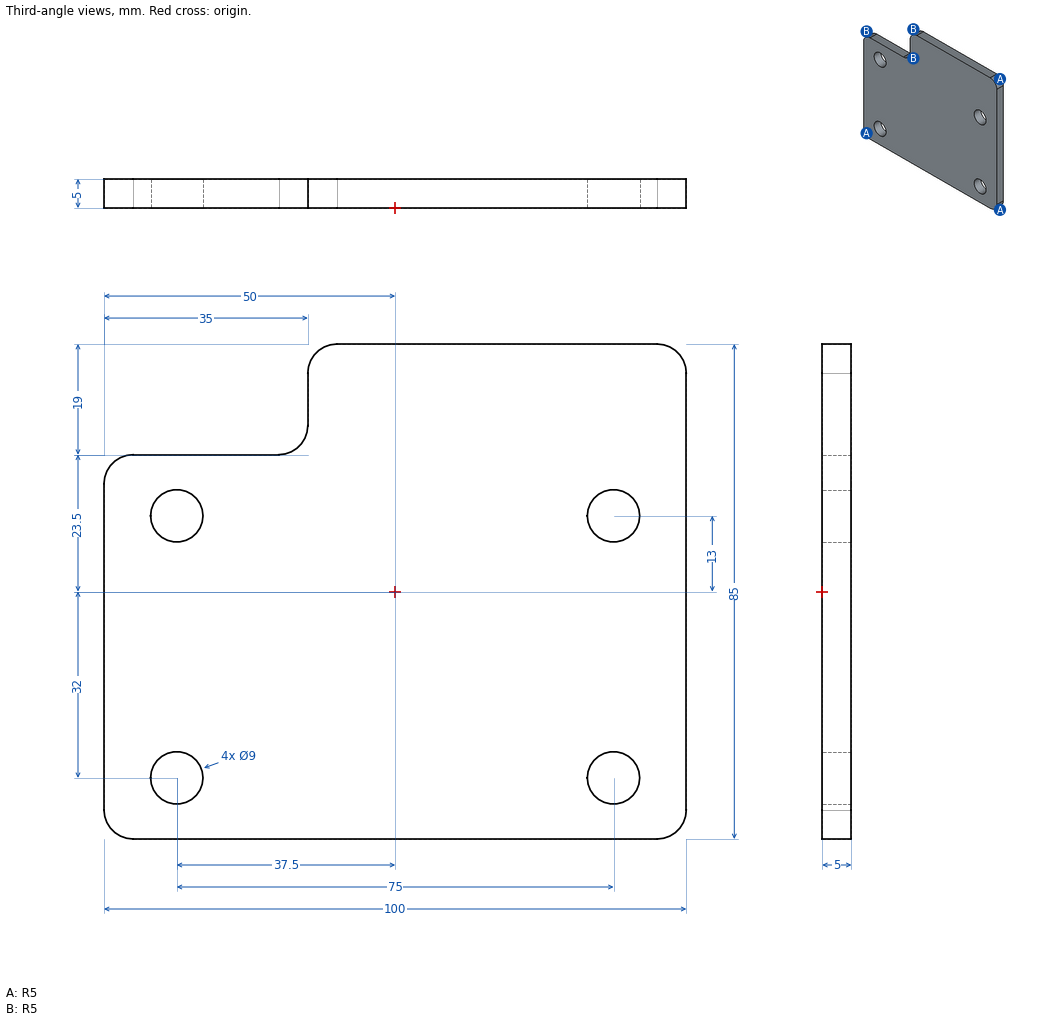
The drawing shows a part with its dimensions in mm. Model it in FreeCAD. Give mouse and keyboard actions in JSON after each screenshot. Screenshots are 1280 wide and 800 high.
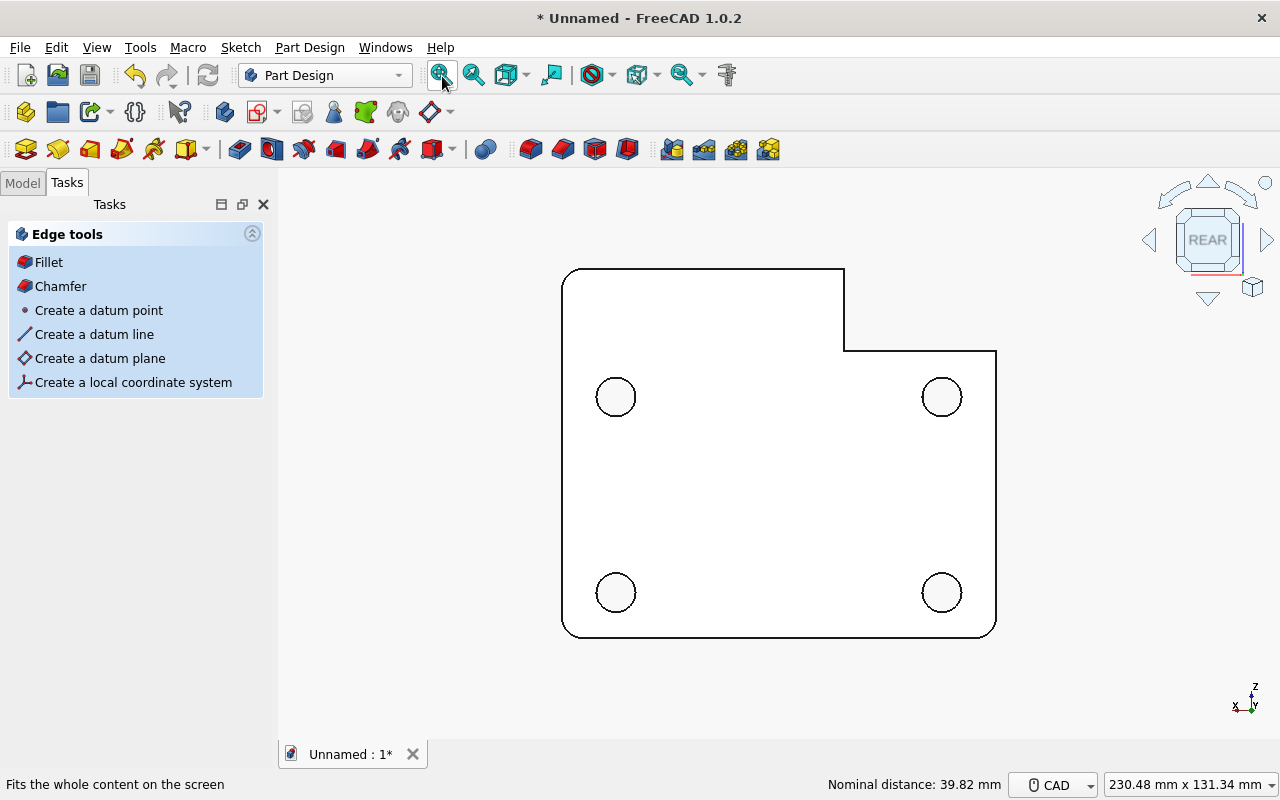
{"action": "scroll", "coordinate": [844, 350], "scroll_direction": "up", "scroll_amount": 4}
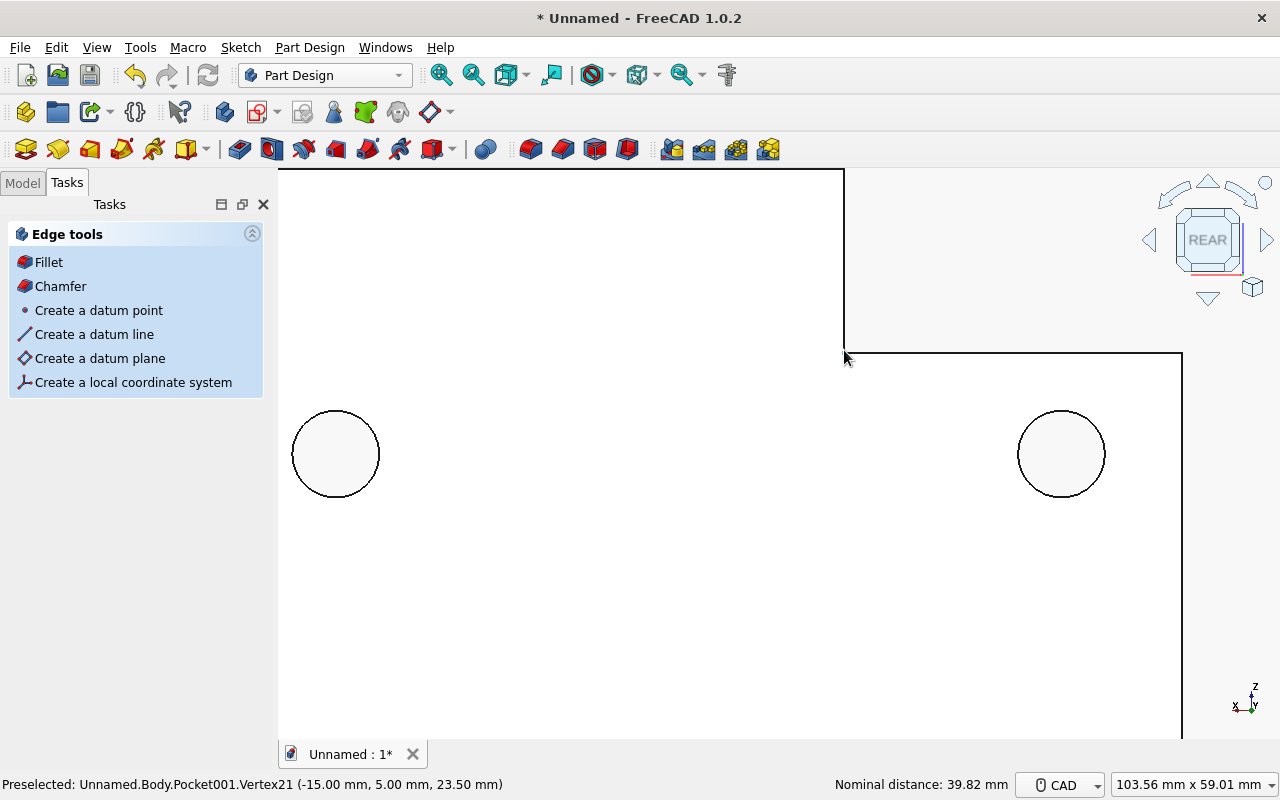
{"action": "key", "text": "v f"}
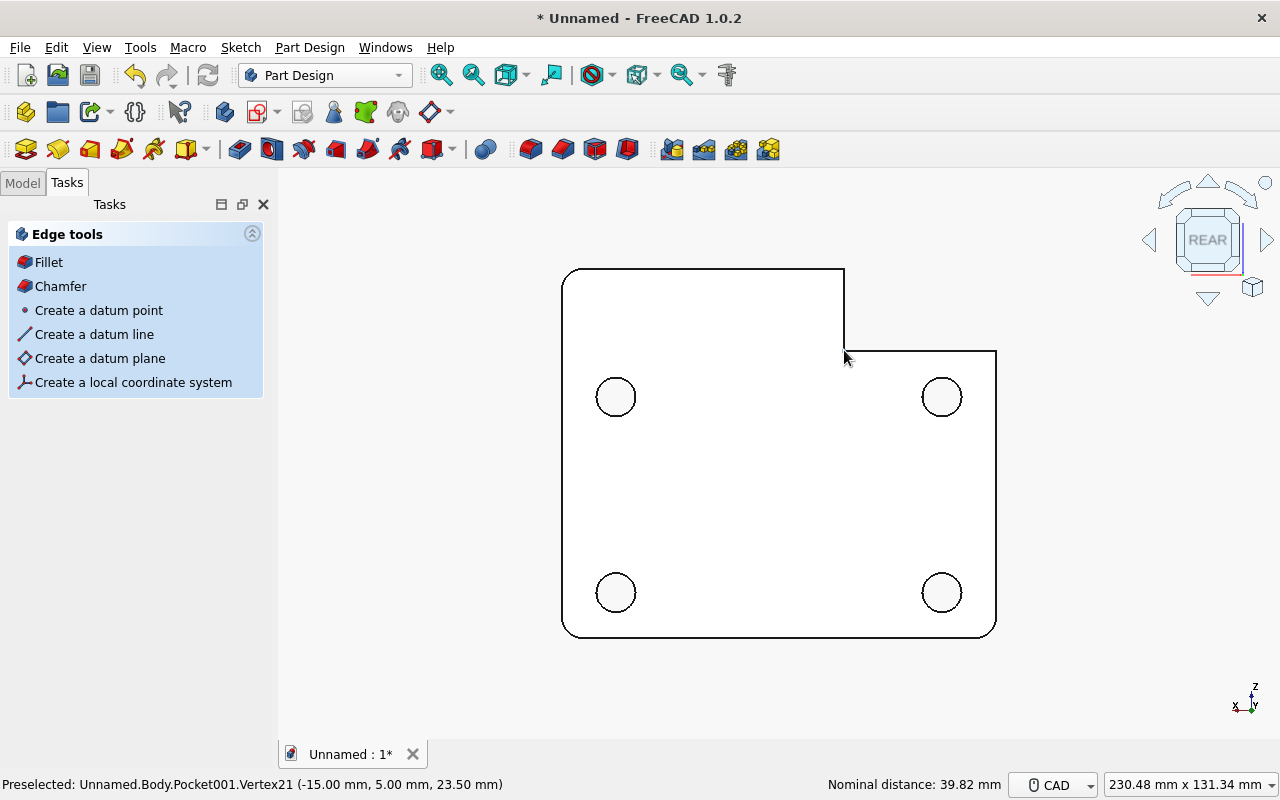
{"action": "key", "text": "6"}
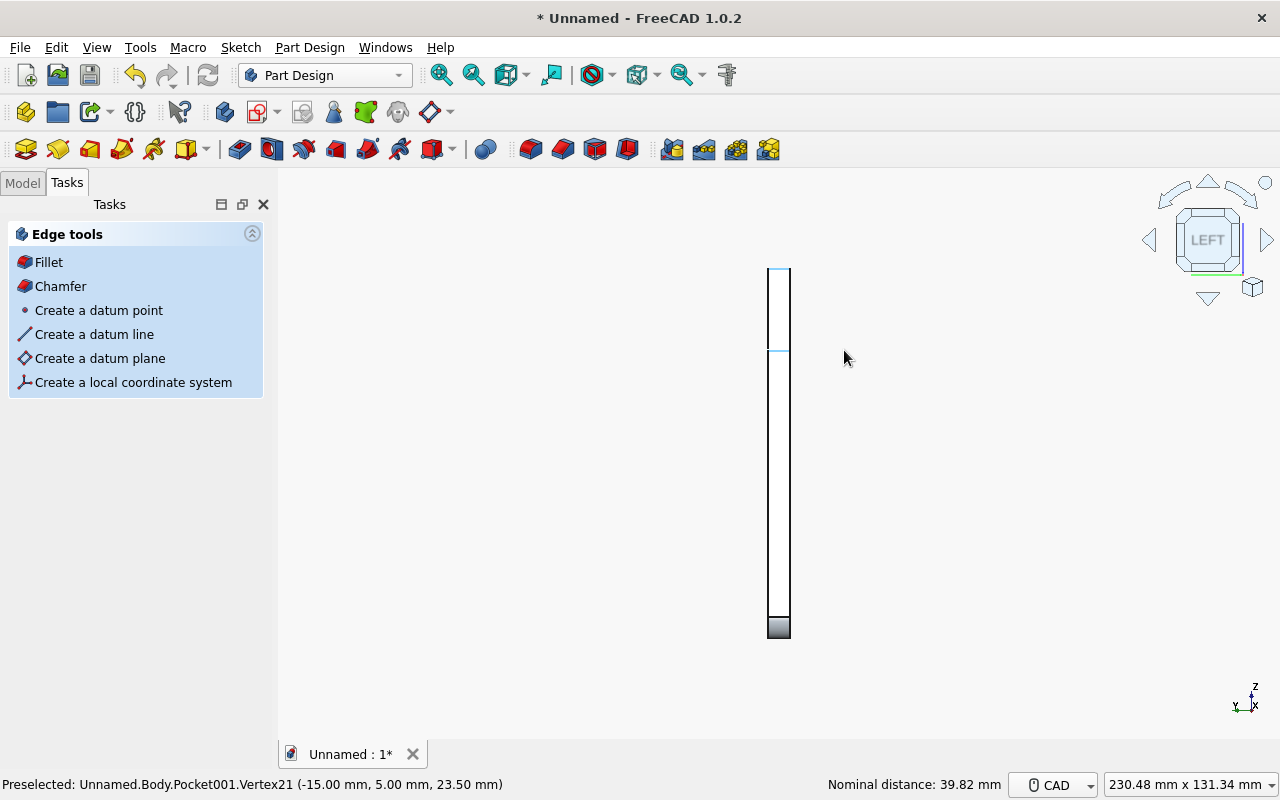
{"action": "scroll", "coordinate": [779, 350], "scroll_direction": "up", "scroll_amount": 4}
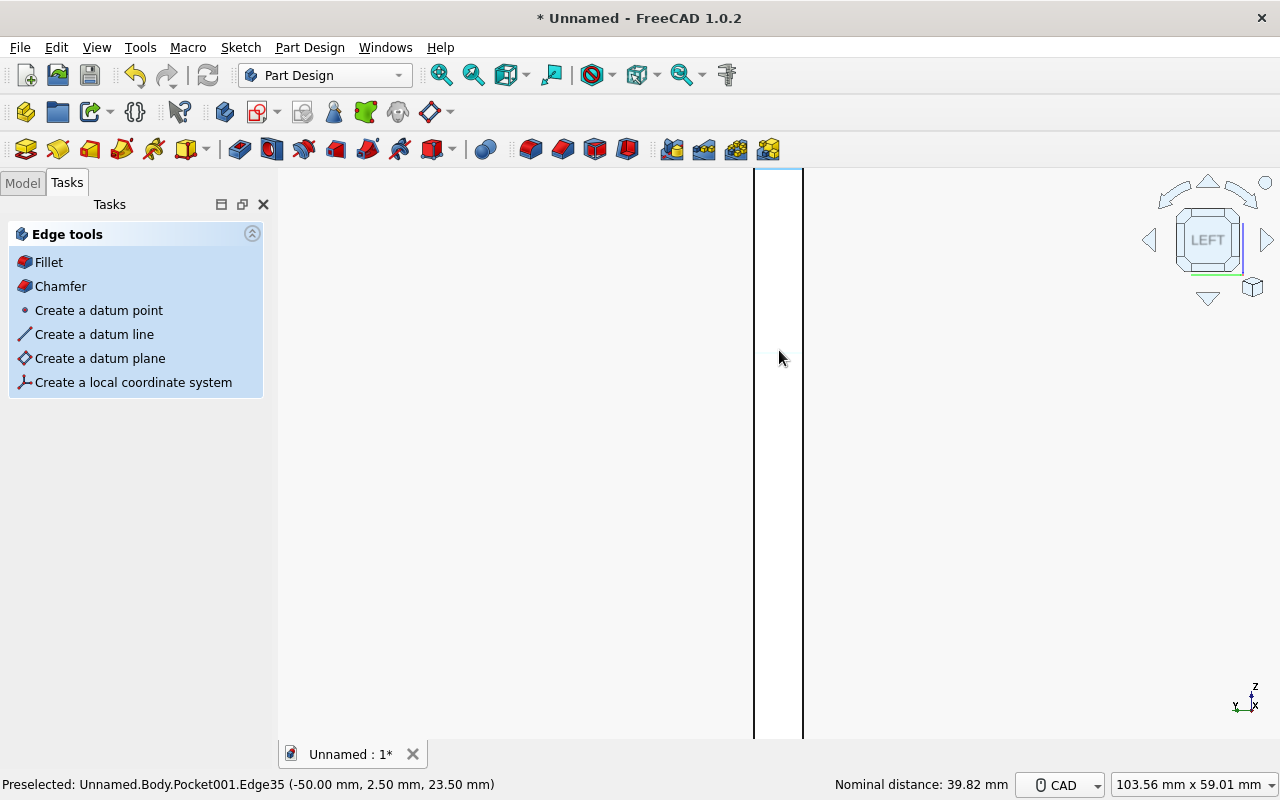
{"action": "key", "text": "v f"}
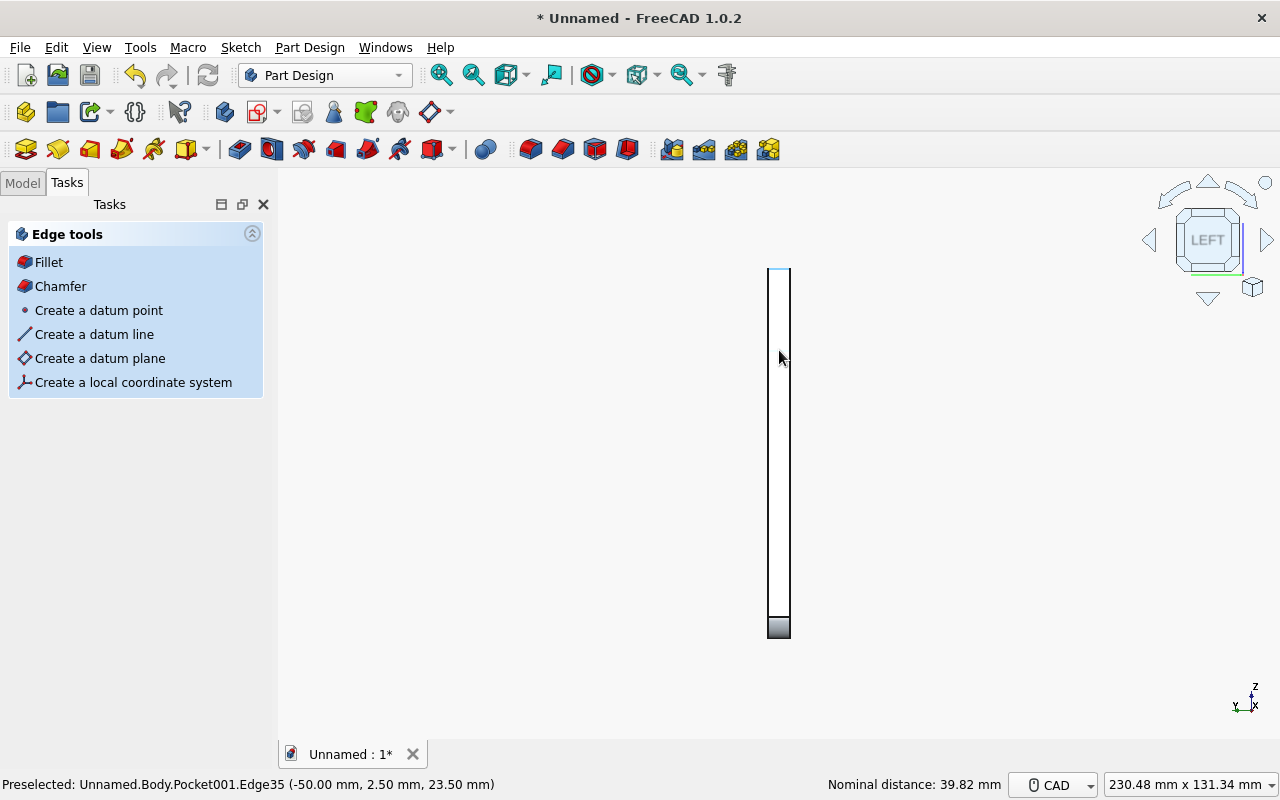
{"action": "key", "text": "v 3"}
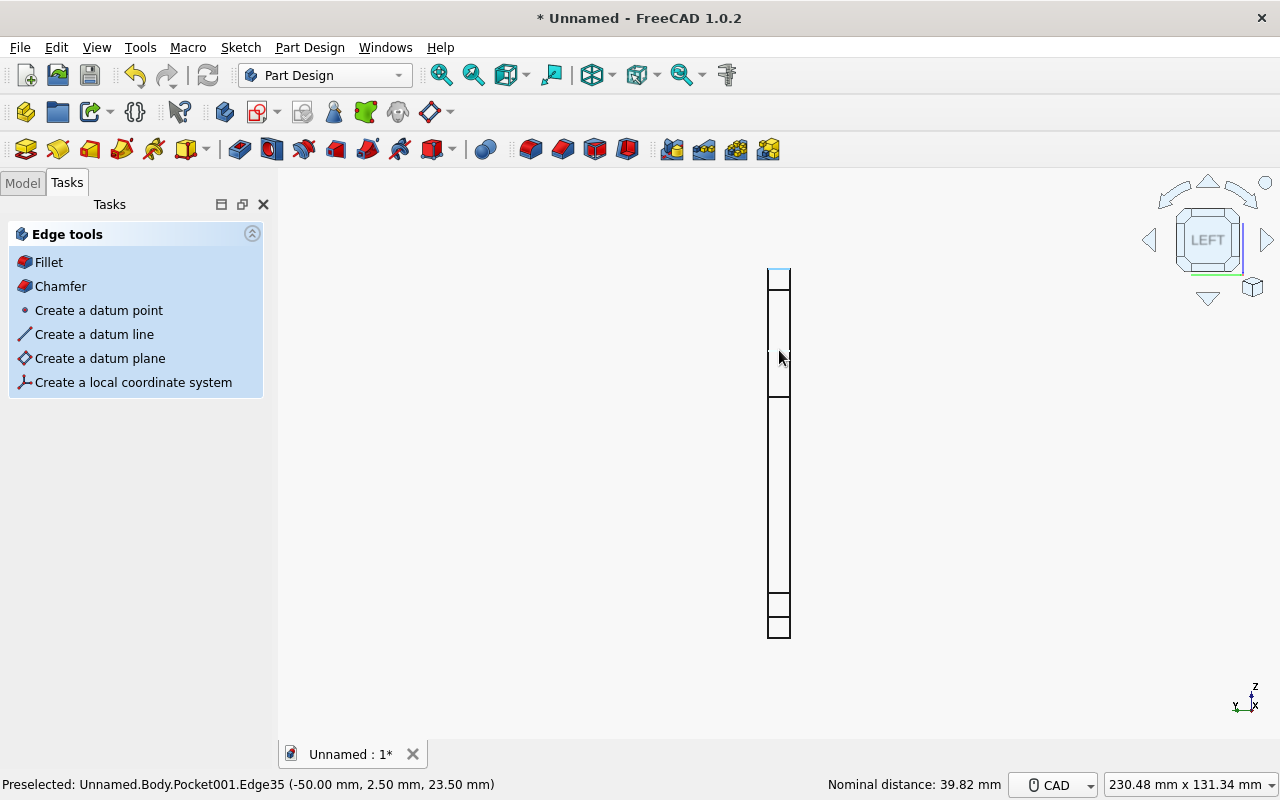
{"action": "key", "text": "0"}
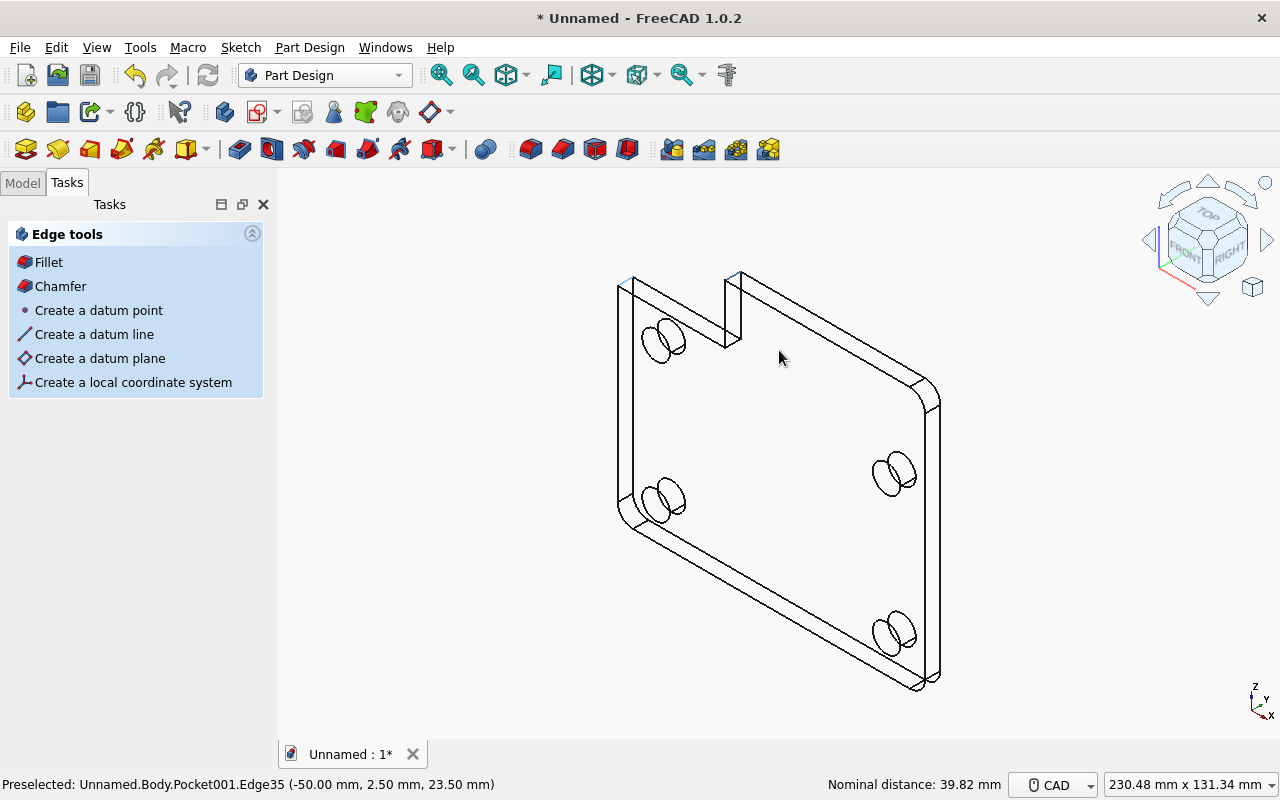
{"action": "left_click", "coordinate": [733, 342], "text": "ctrl"}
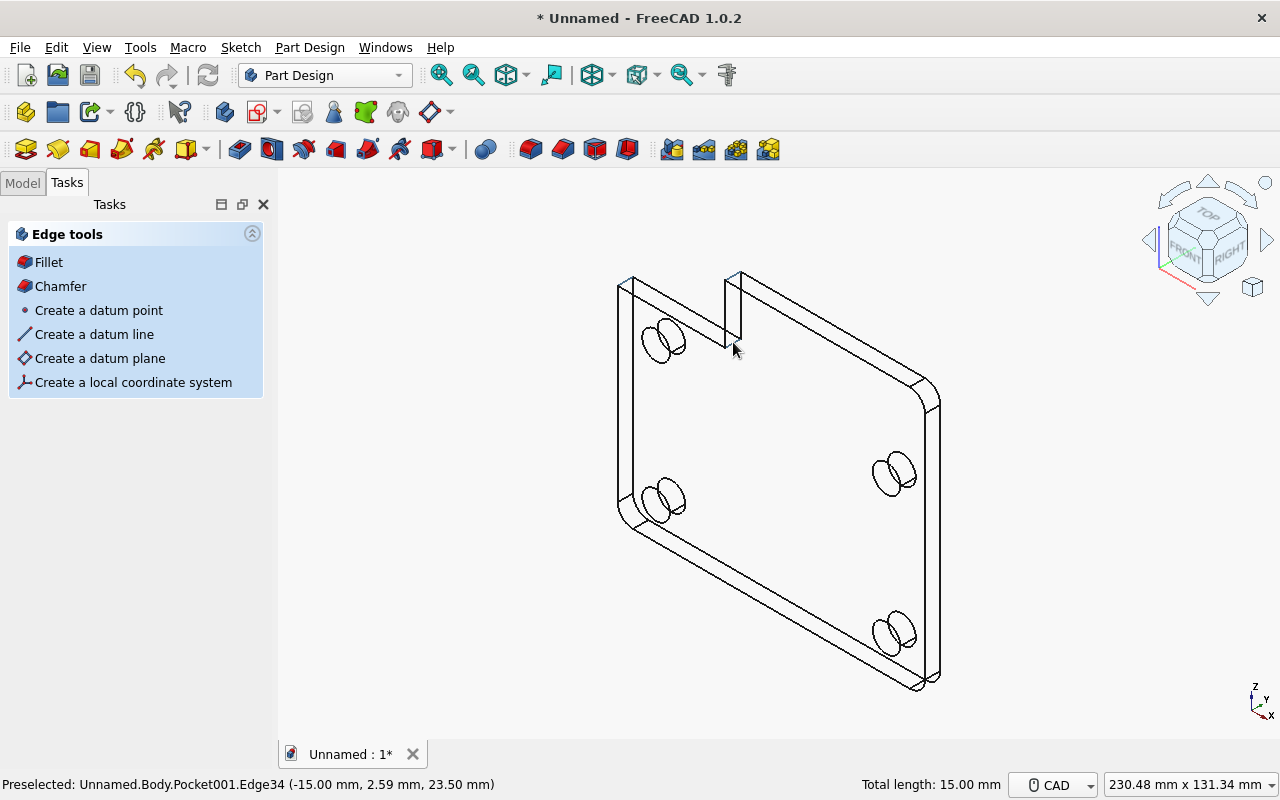
{"action": "key", "text": "v 1"}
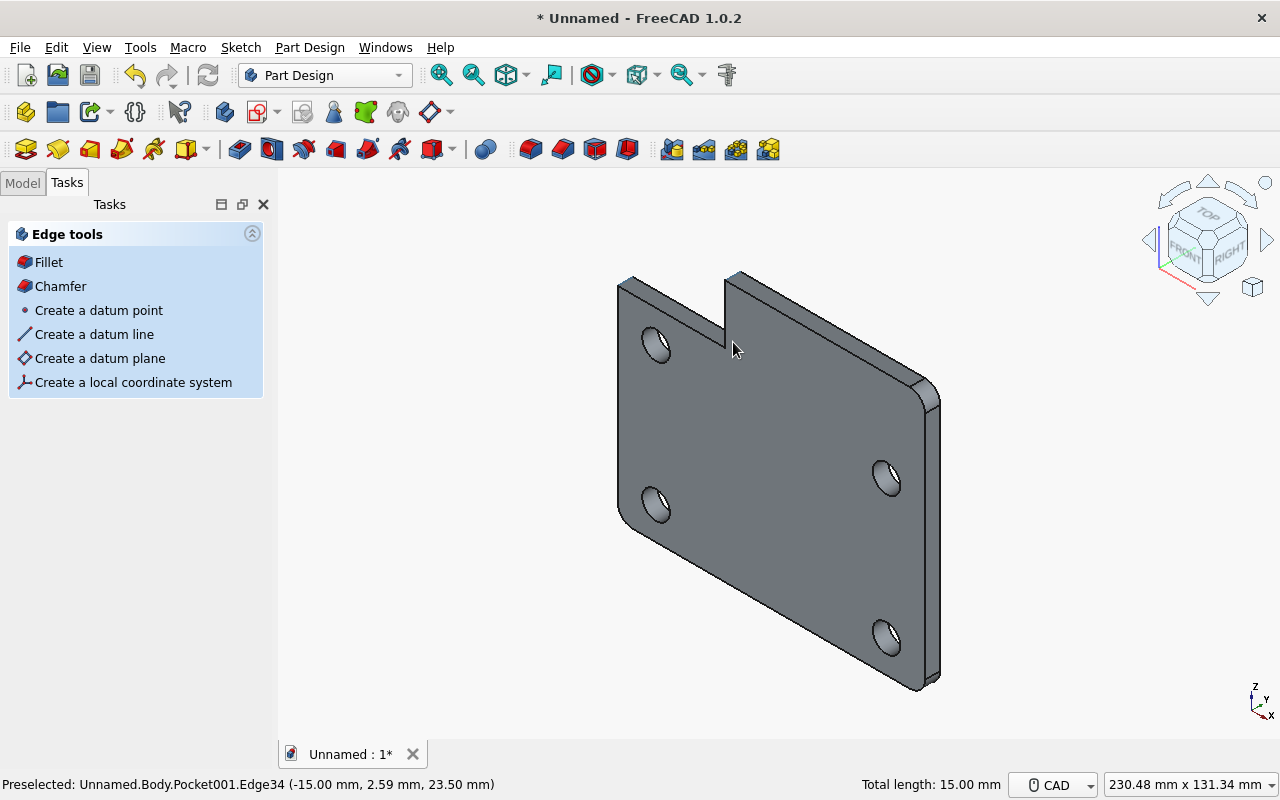
{"action": "left_click", "coordinate": [532, 150]}